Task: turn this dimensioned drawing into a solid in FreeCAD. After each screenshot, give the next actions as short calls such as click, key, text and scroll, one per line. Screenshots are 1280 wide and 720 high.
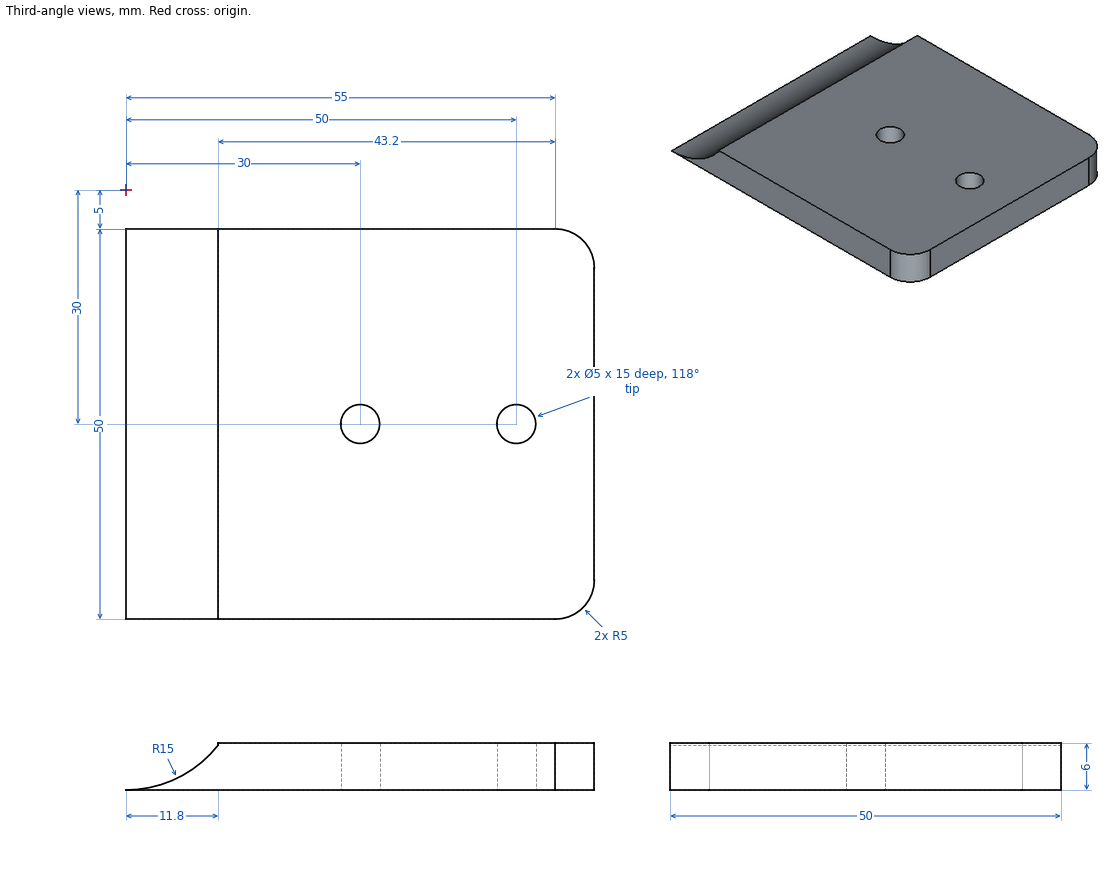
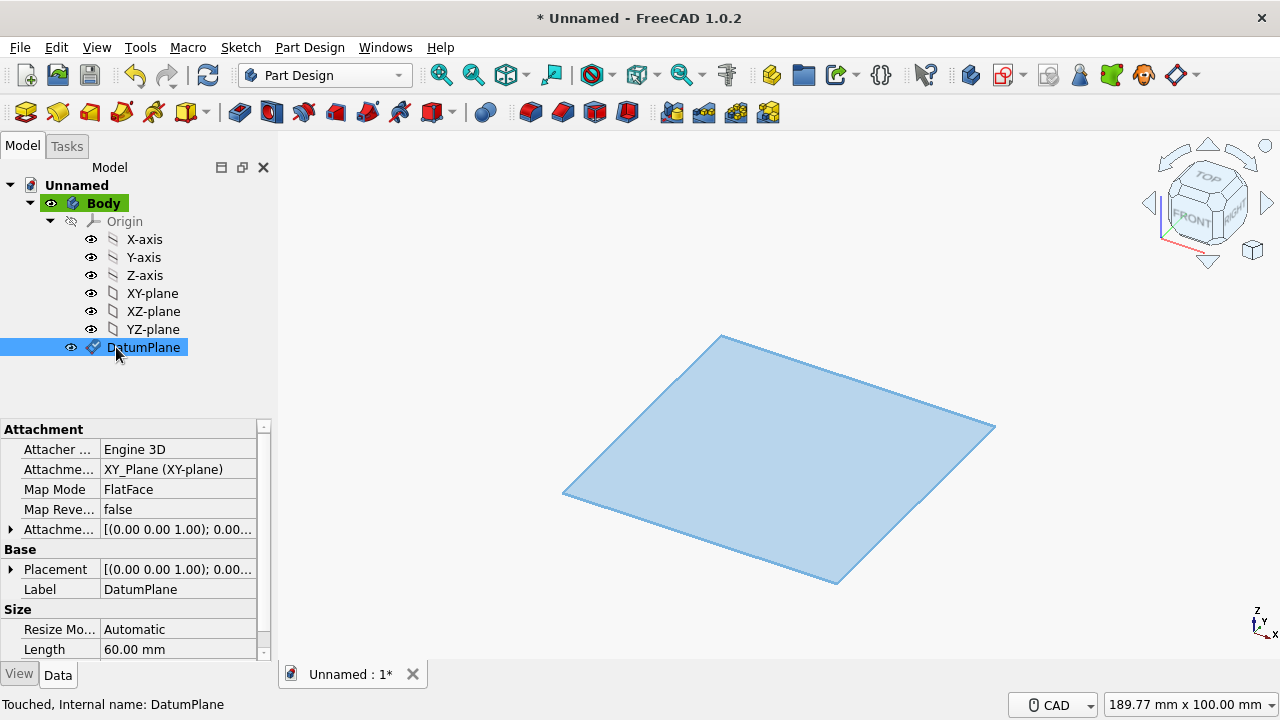
click(1004, 76)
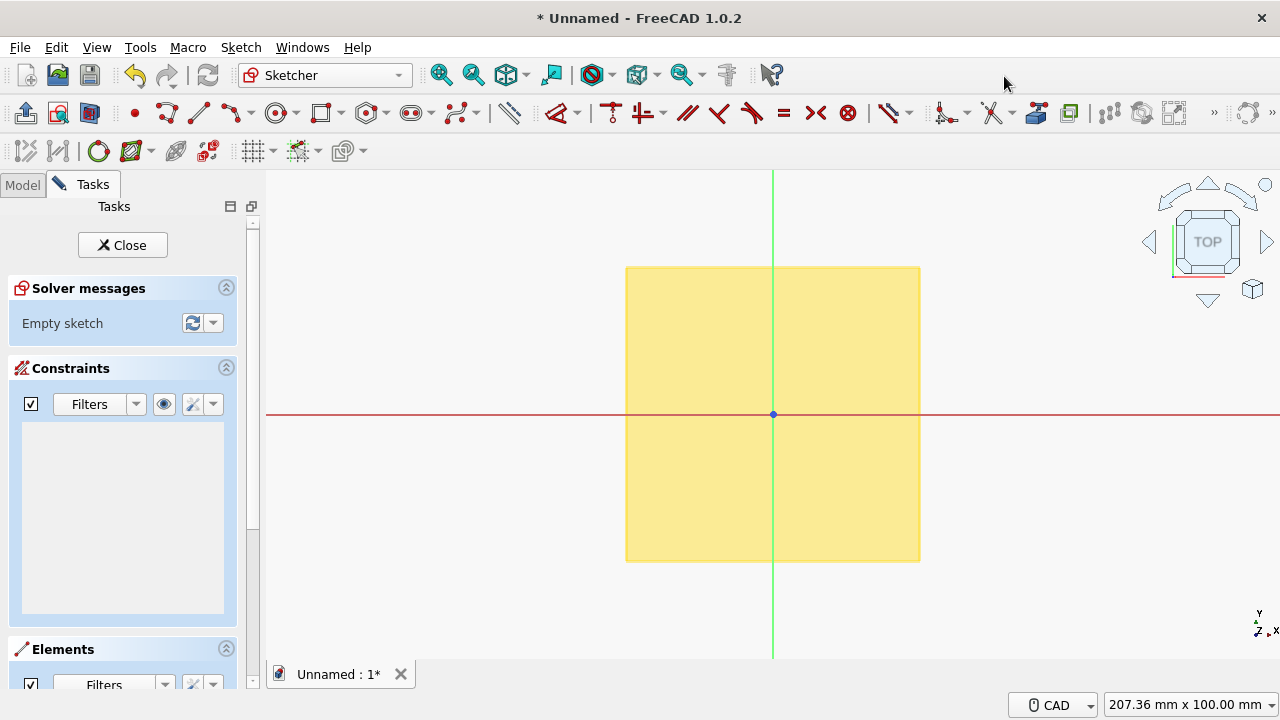
scroll(294, 198, down, 1)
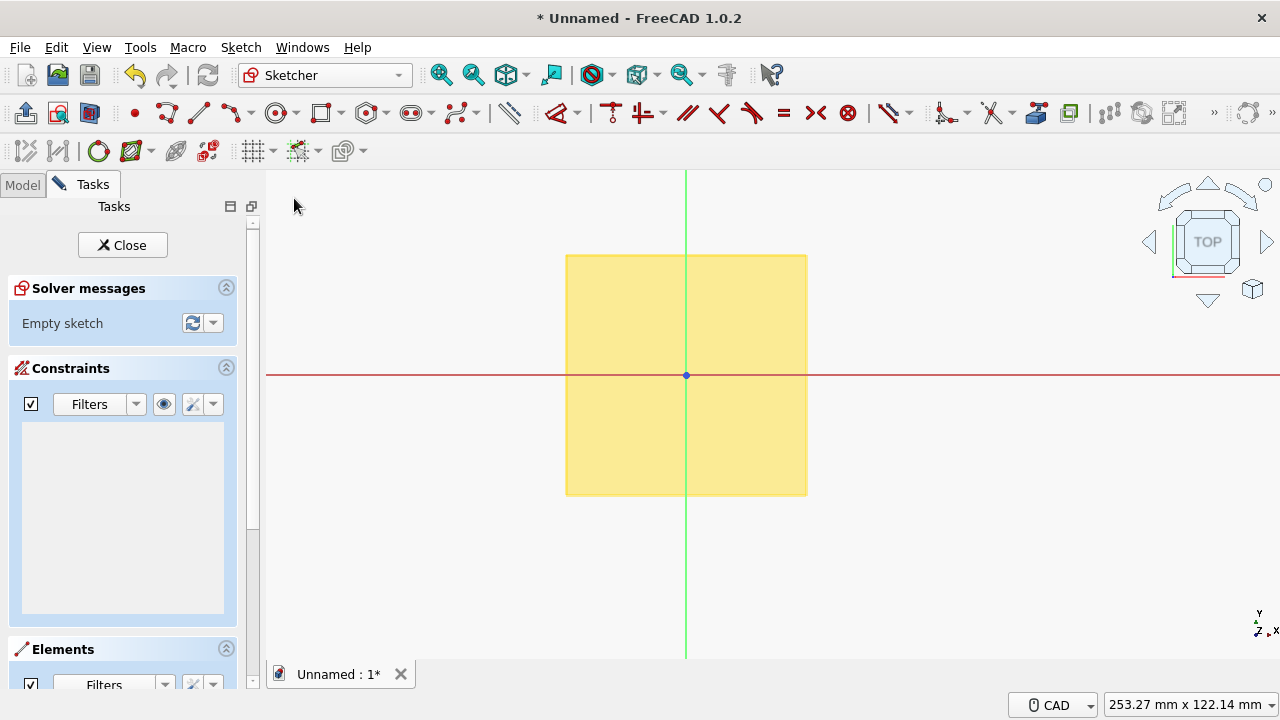
scroll(1013, 629, up, 2)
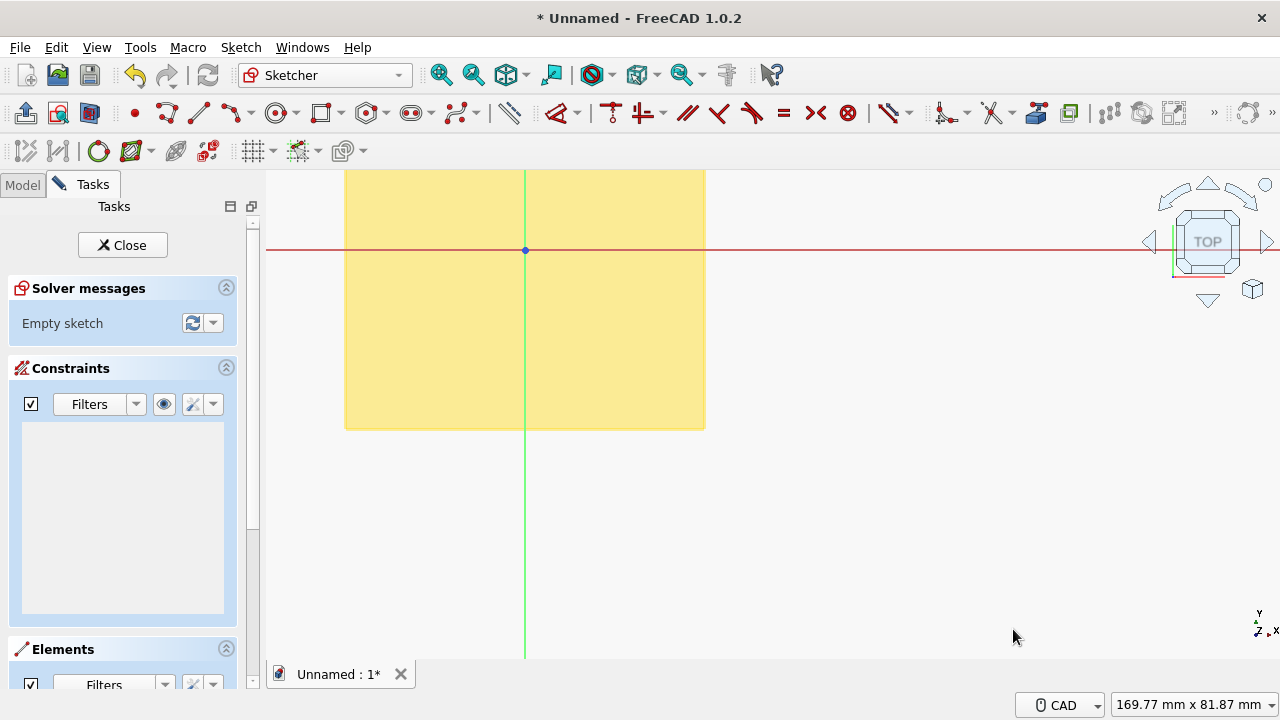
click(168, 114)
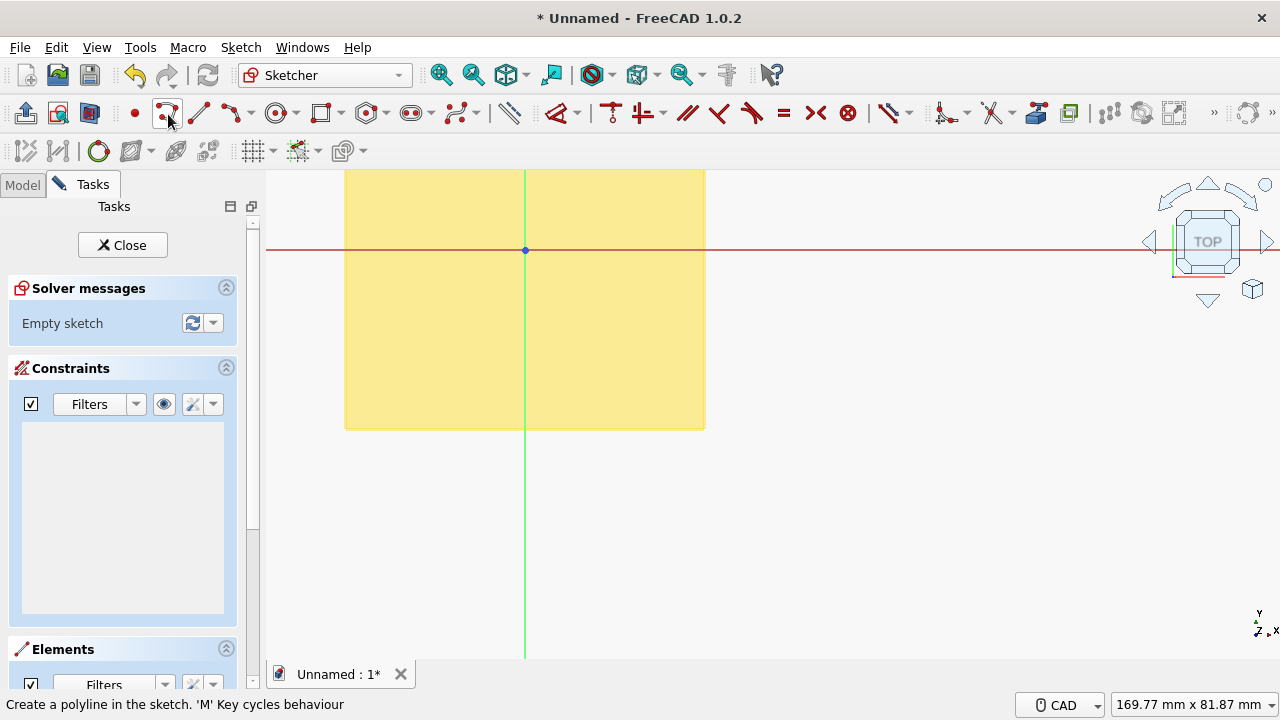
click(854, 280)
click(596, 280)
click(596, 579)
click(854, 579)
right_click(854, 579)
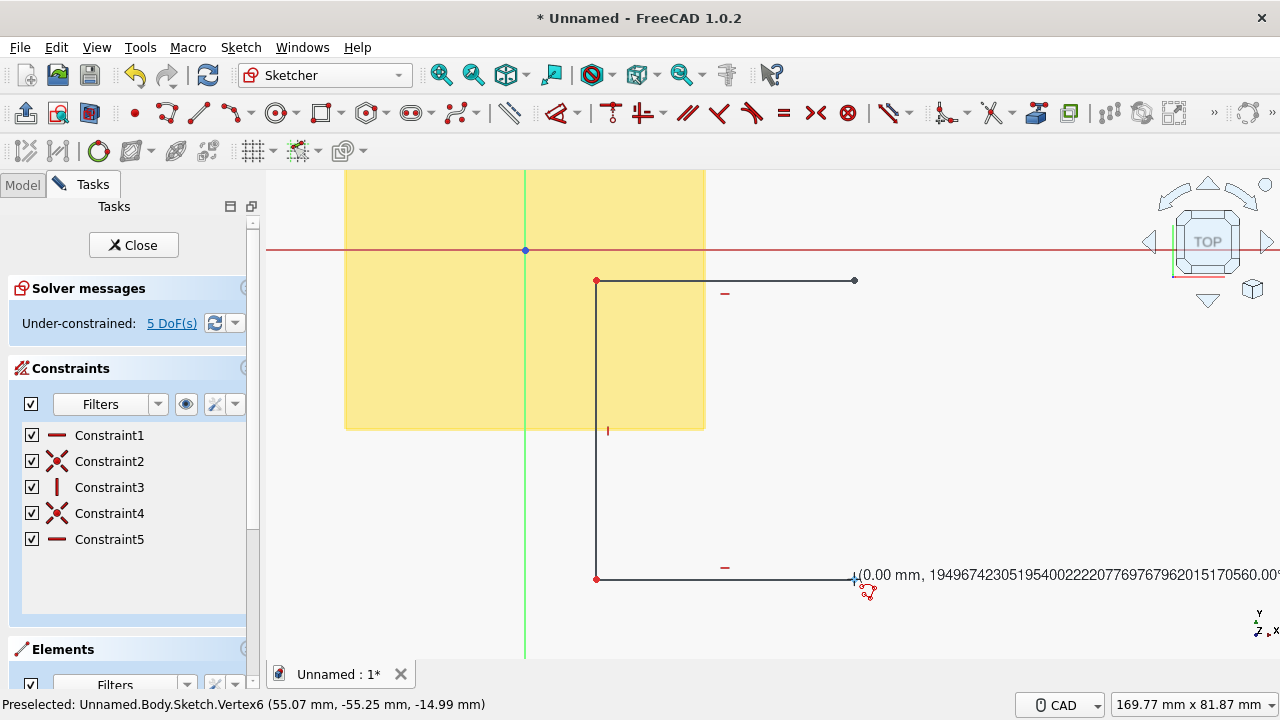
click(200, 114)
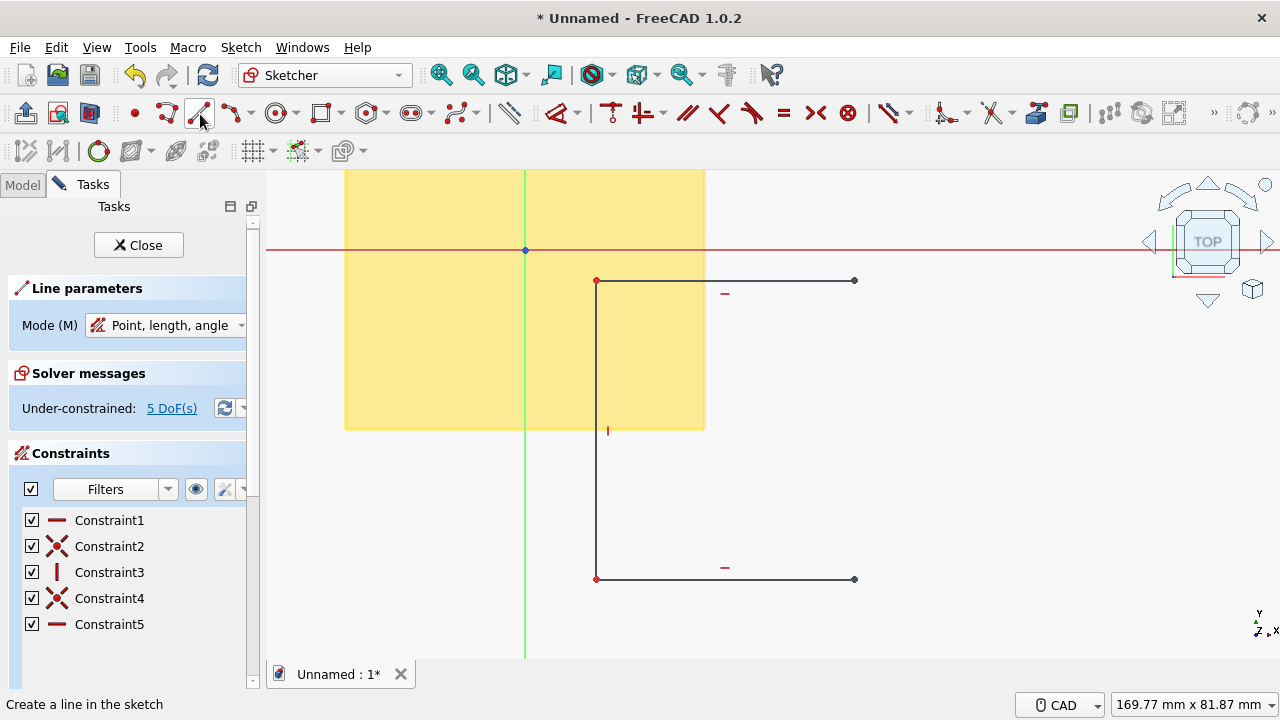
click(883, 549)
click(883, 310)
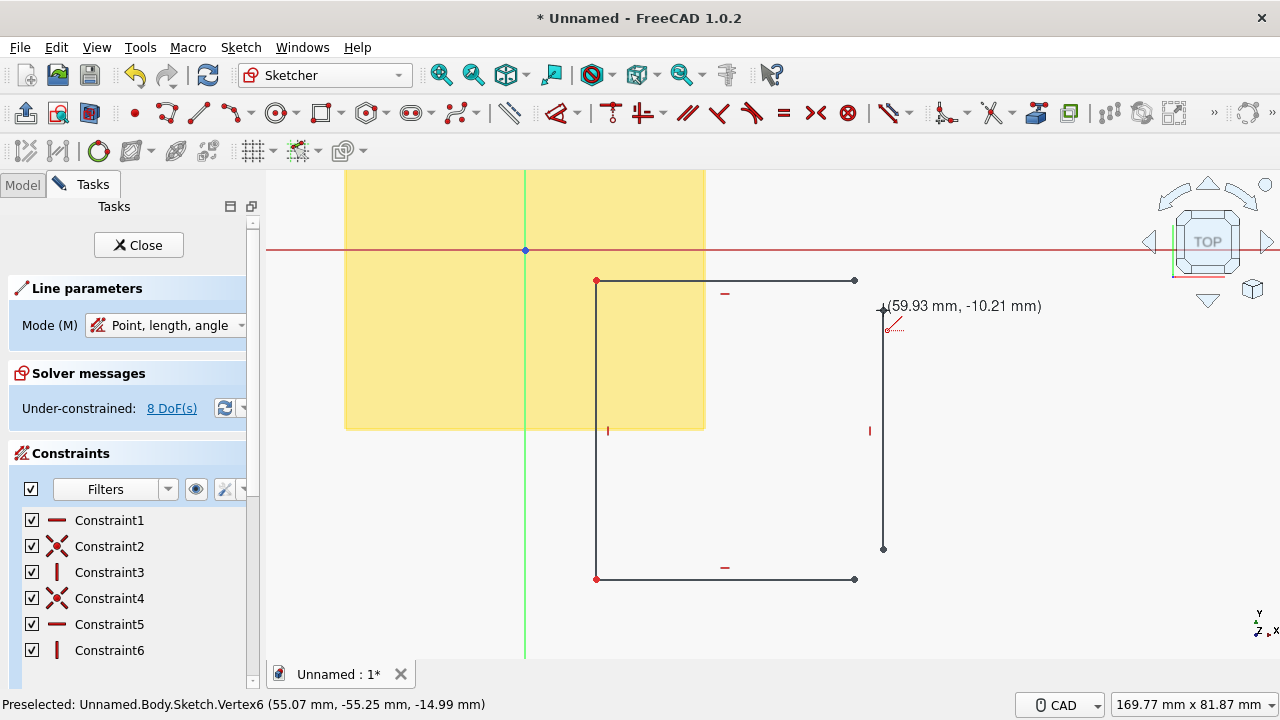
click(232, 114)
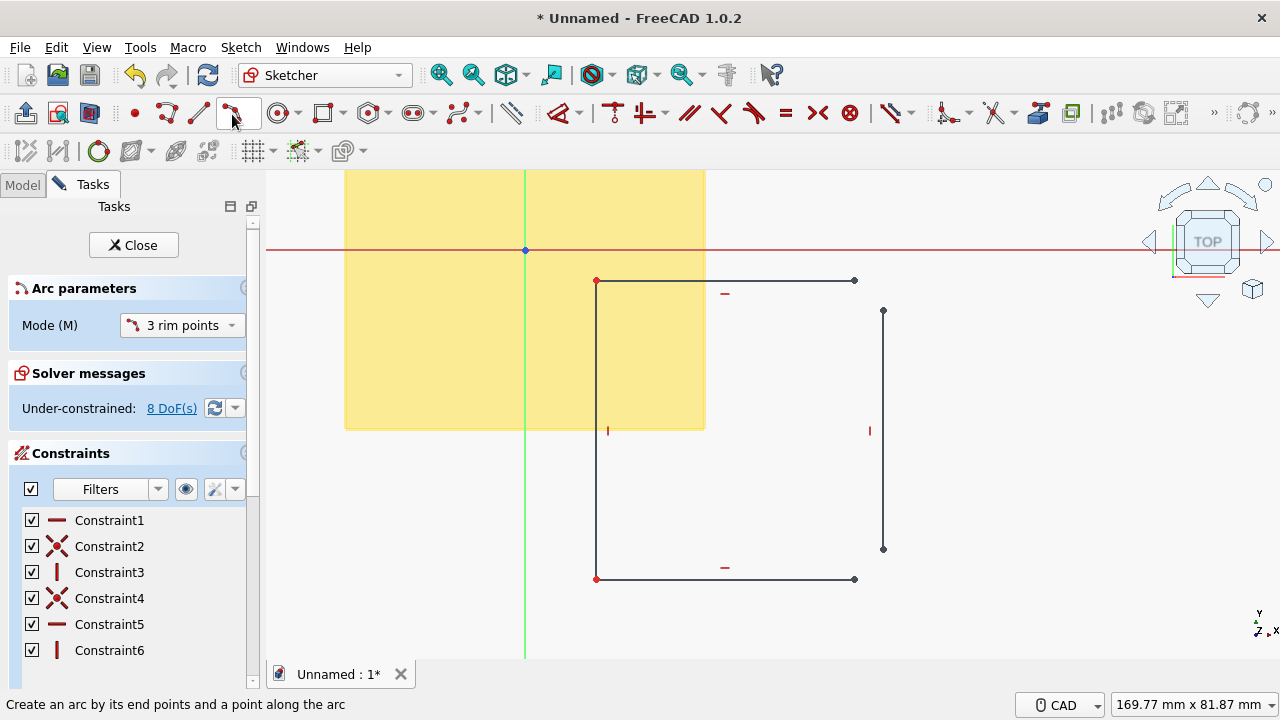
click(854, 580)
click(883, 550)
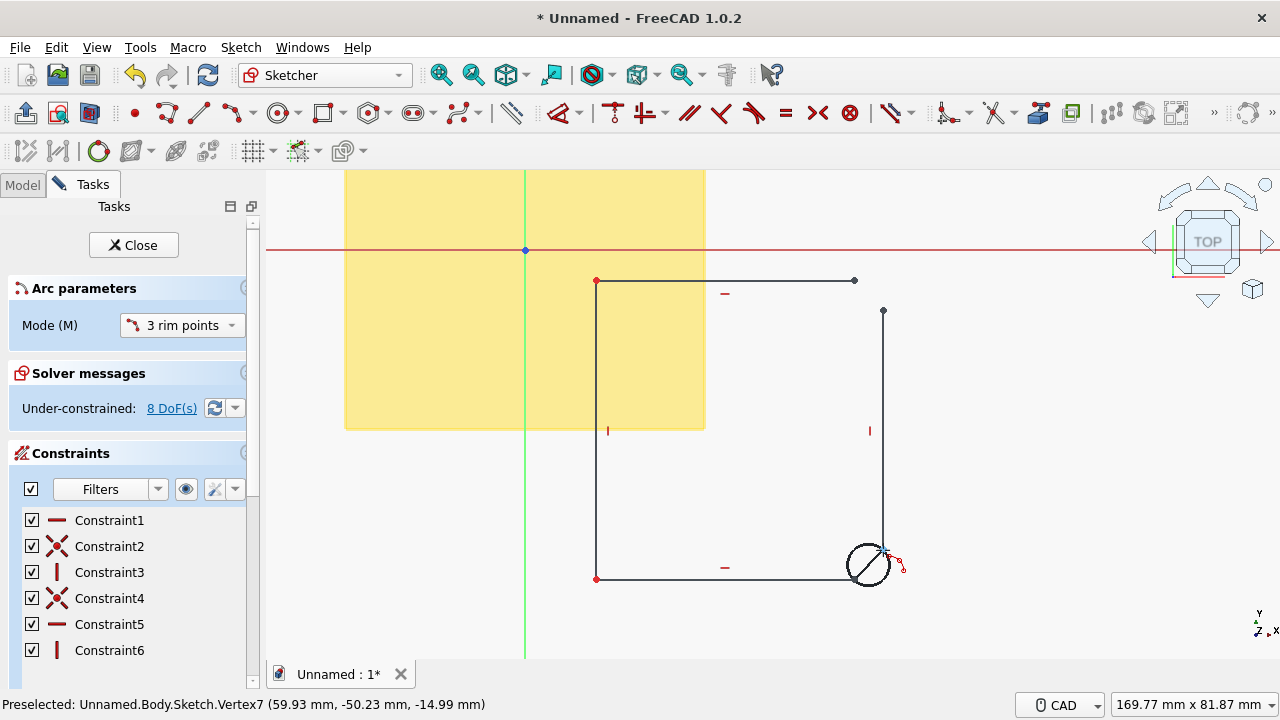
scroll(875, 570, up, 3)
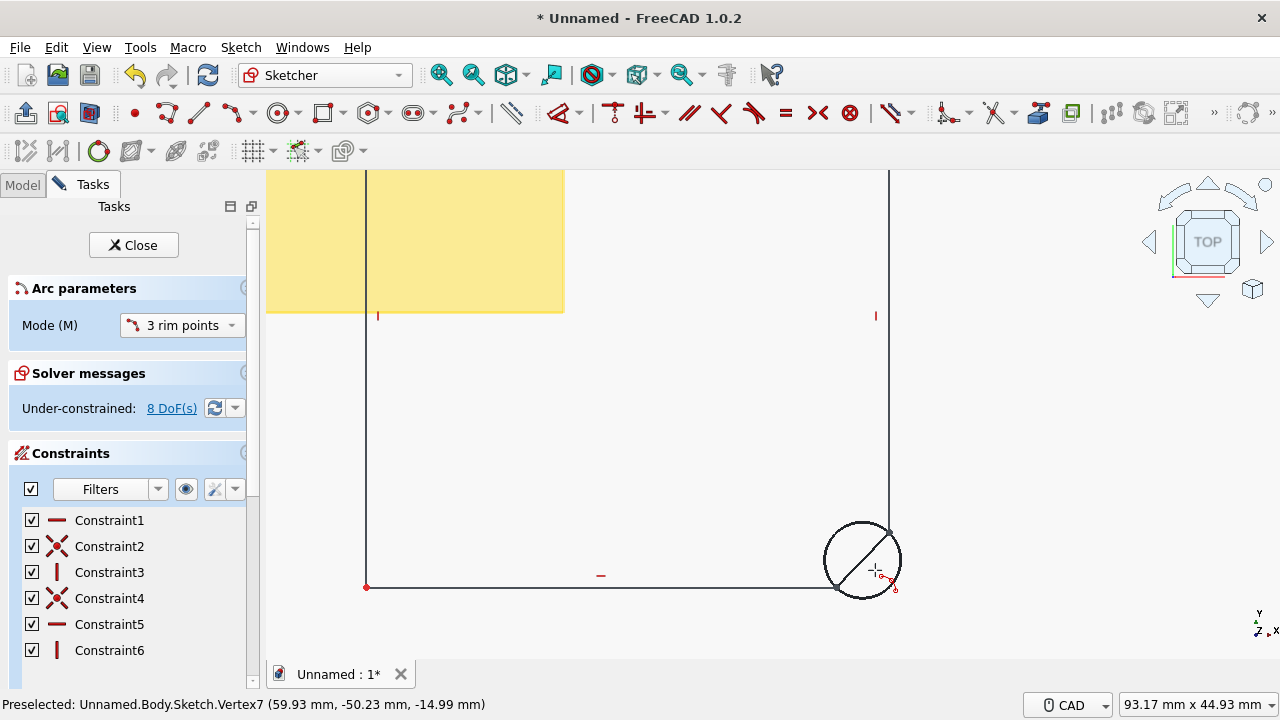
click(874, 569)